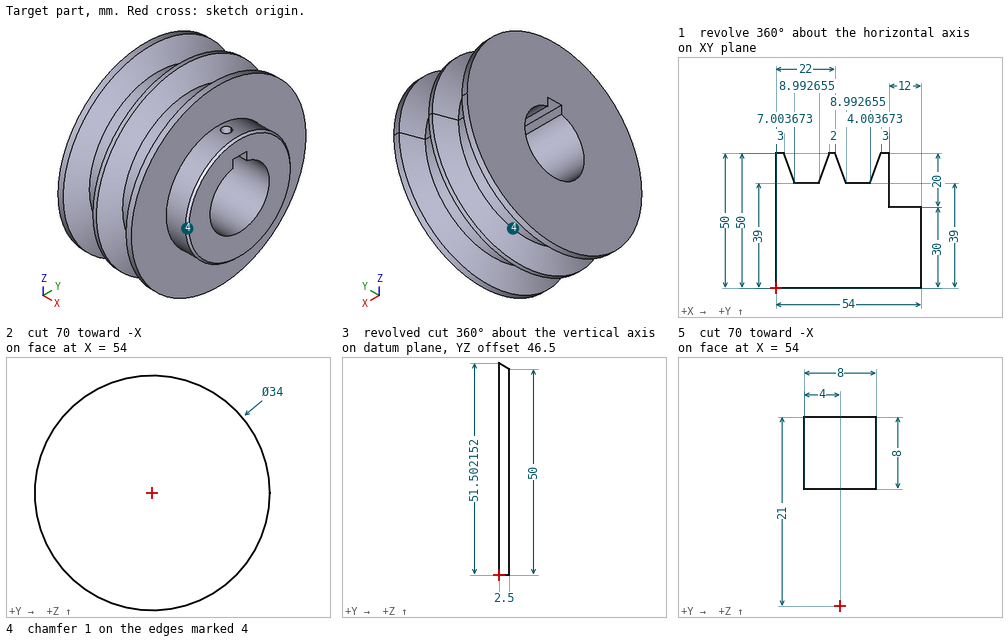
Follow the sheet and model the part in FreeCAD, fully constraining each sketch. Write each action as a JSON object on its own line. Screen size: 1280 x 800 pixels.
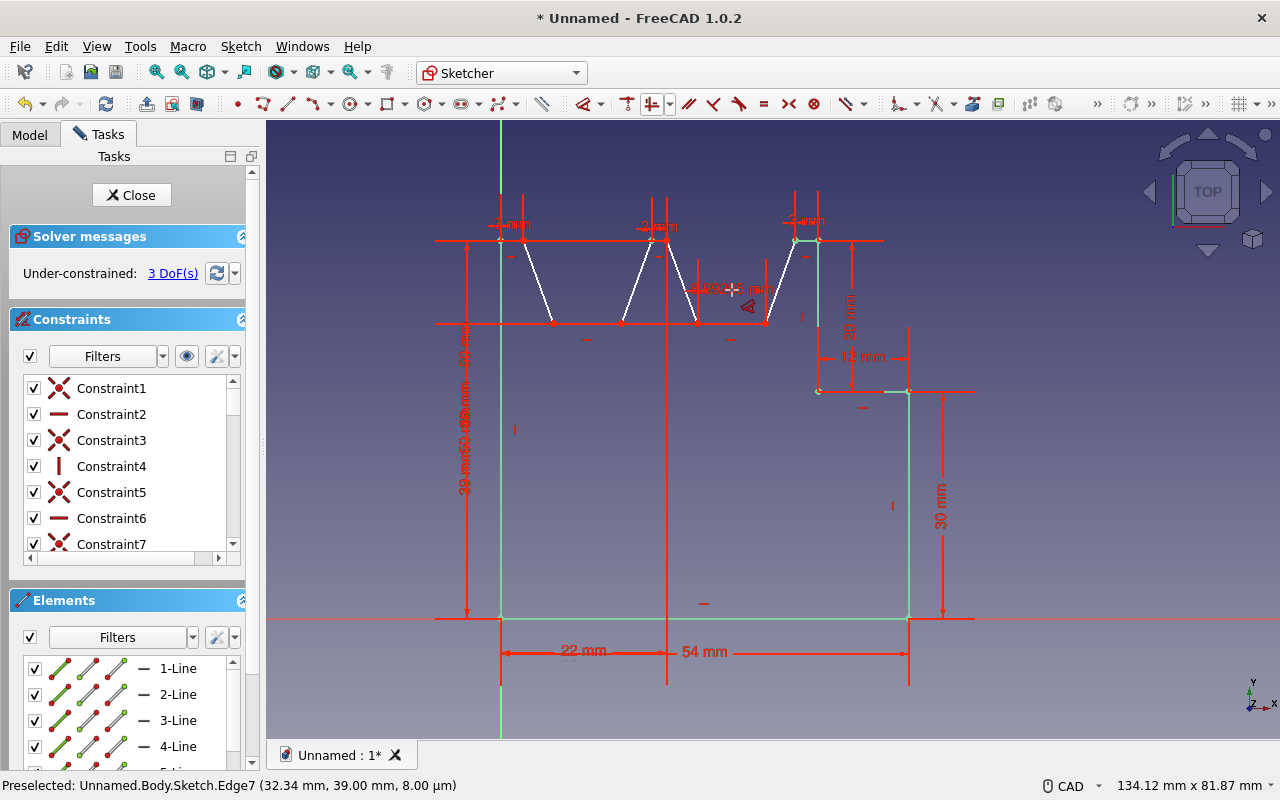
{"action": "left_click", "coordinate": [601, 324]}
{"action": "left_click", "coordinate": [588, 290]}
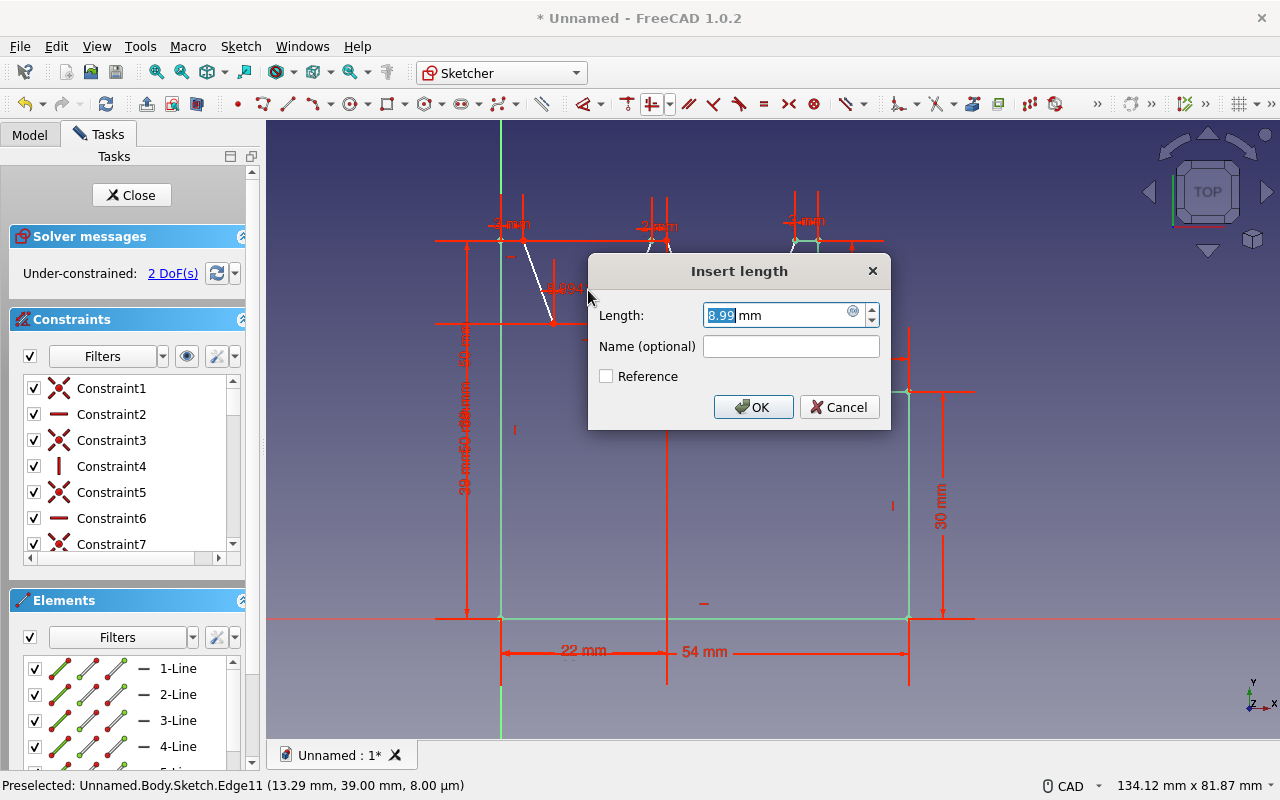
{"action": "type", "text": "8.992655"}
{"action": "key", "text": "Return"}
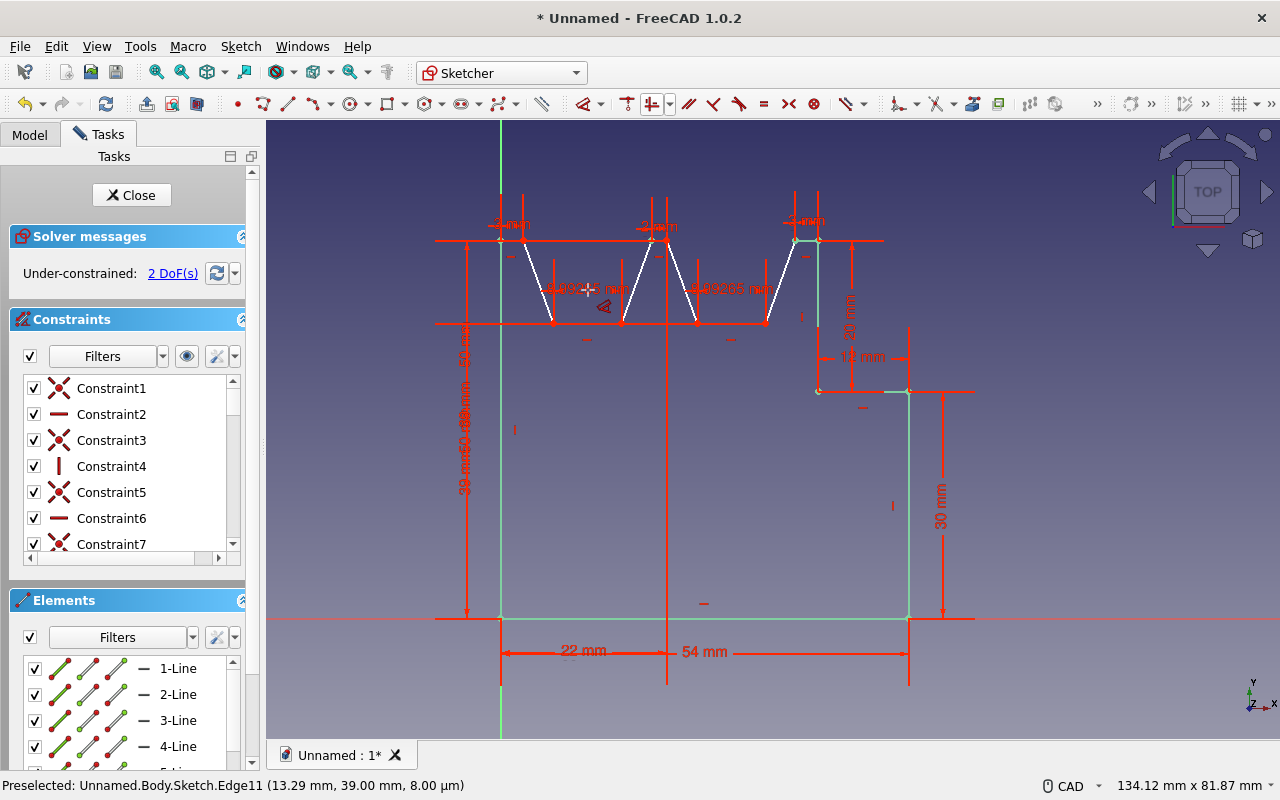
{"action": "left_click", "coordinate": [554, 324]}
{"action": "left_click", "coordinate": [515, 290]}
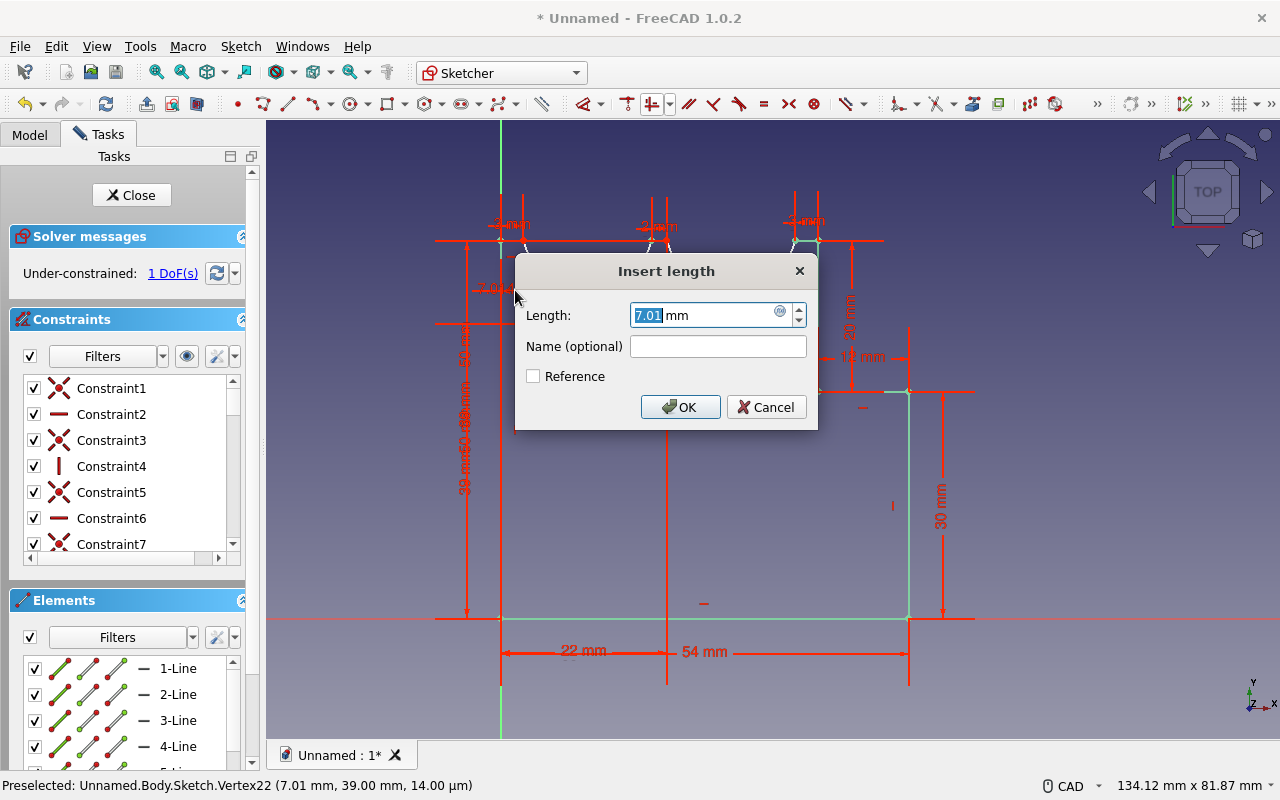
{"action": "type", "text": "7.003673"}
{"action": "key", "text": "Return"}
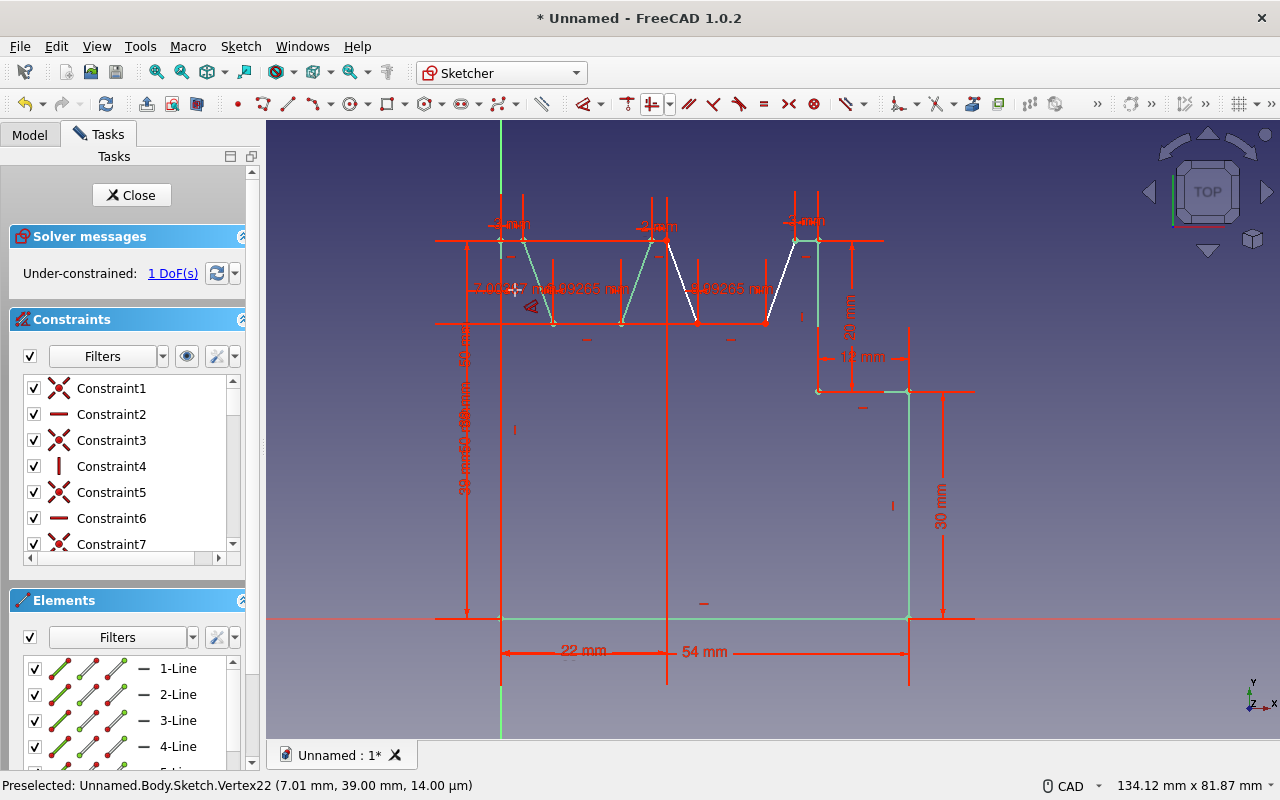
{"action": "scroll", "coordinate": [786, 266], "scroll_direction": "up", "scroll_amount": 2}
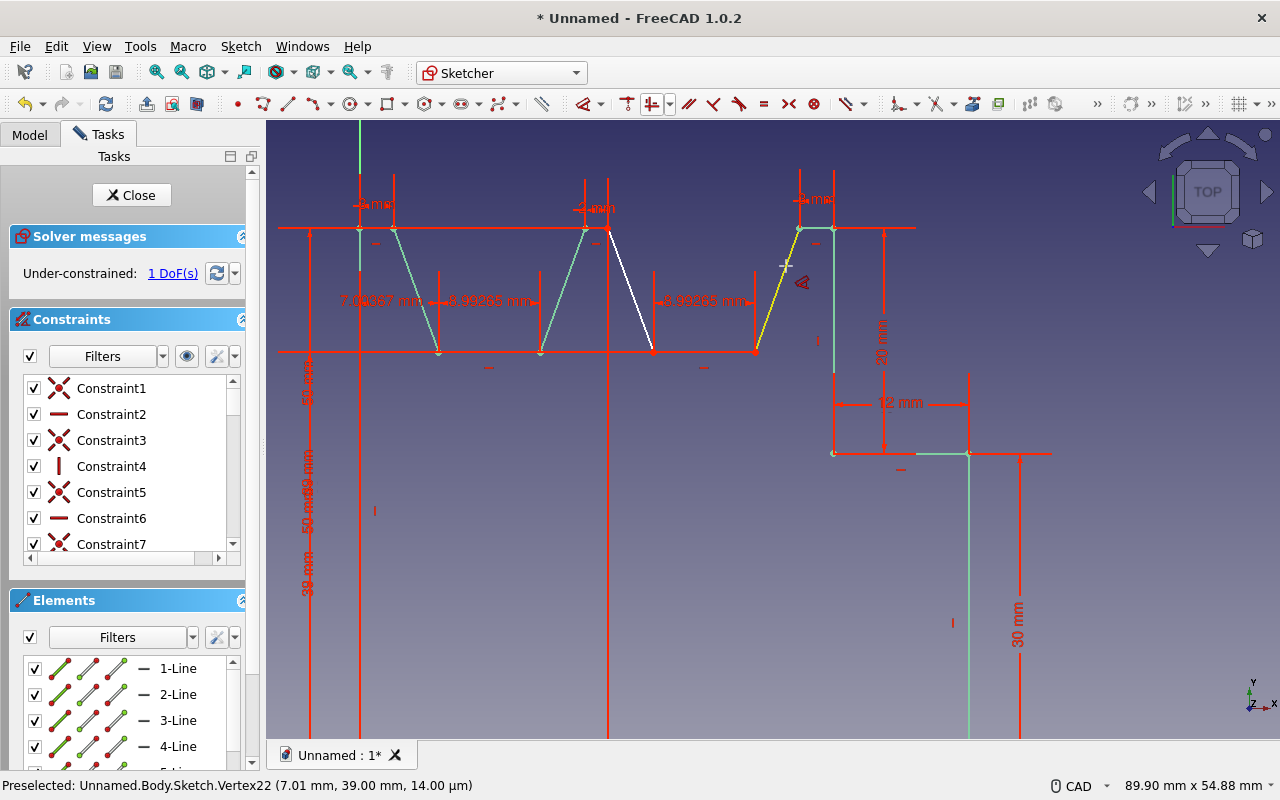
{"action": "left_click", "coordinate": [786, 265]}
{"action": "left_click", "coordinate": [777, 386]}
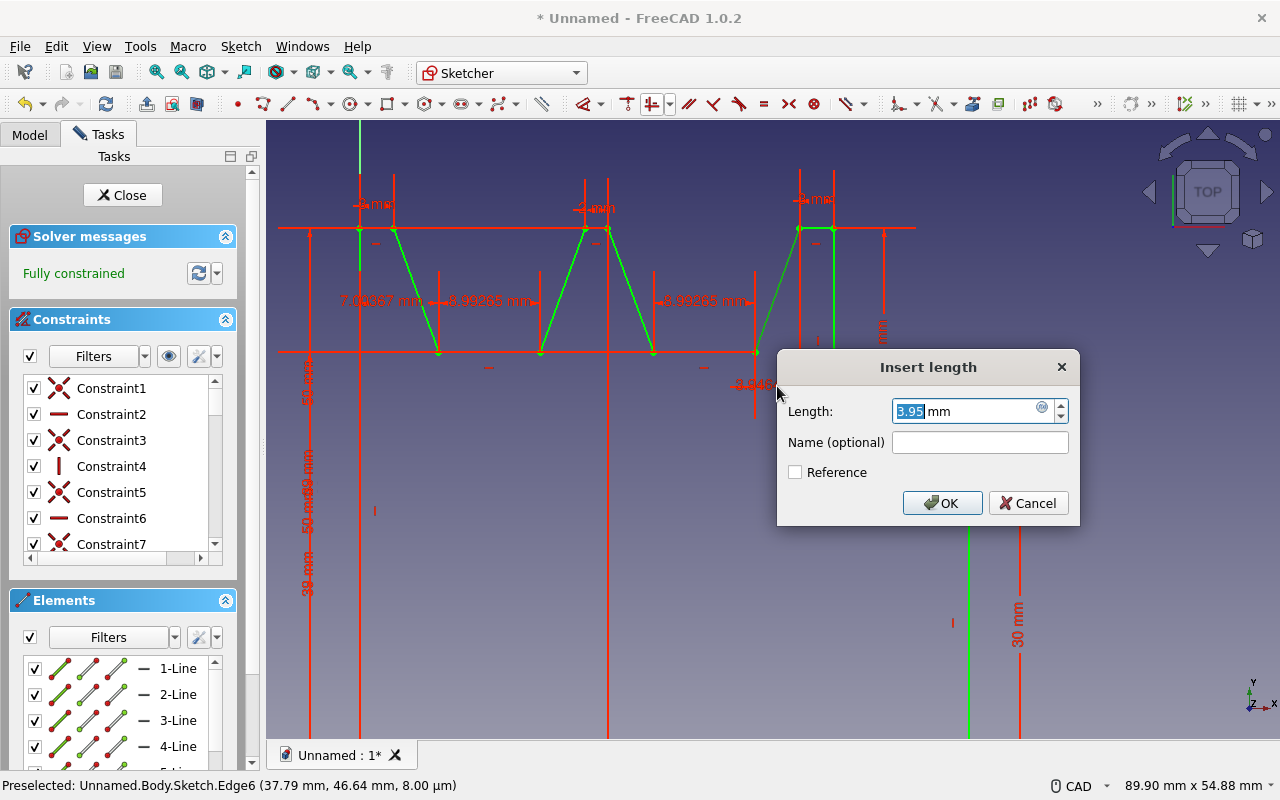
{"action": "type", "text": "4.003673"}
{"action": "key", "text": "Return"}
{"action": "key", "text": "Escape"}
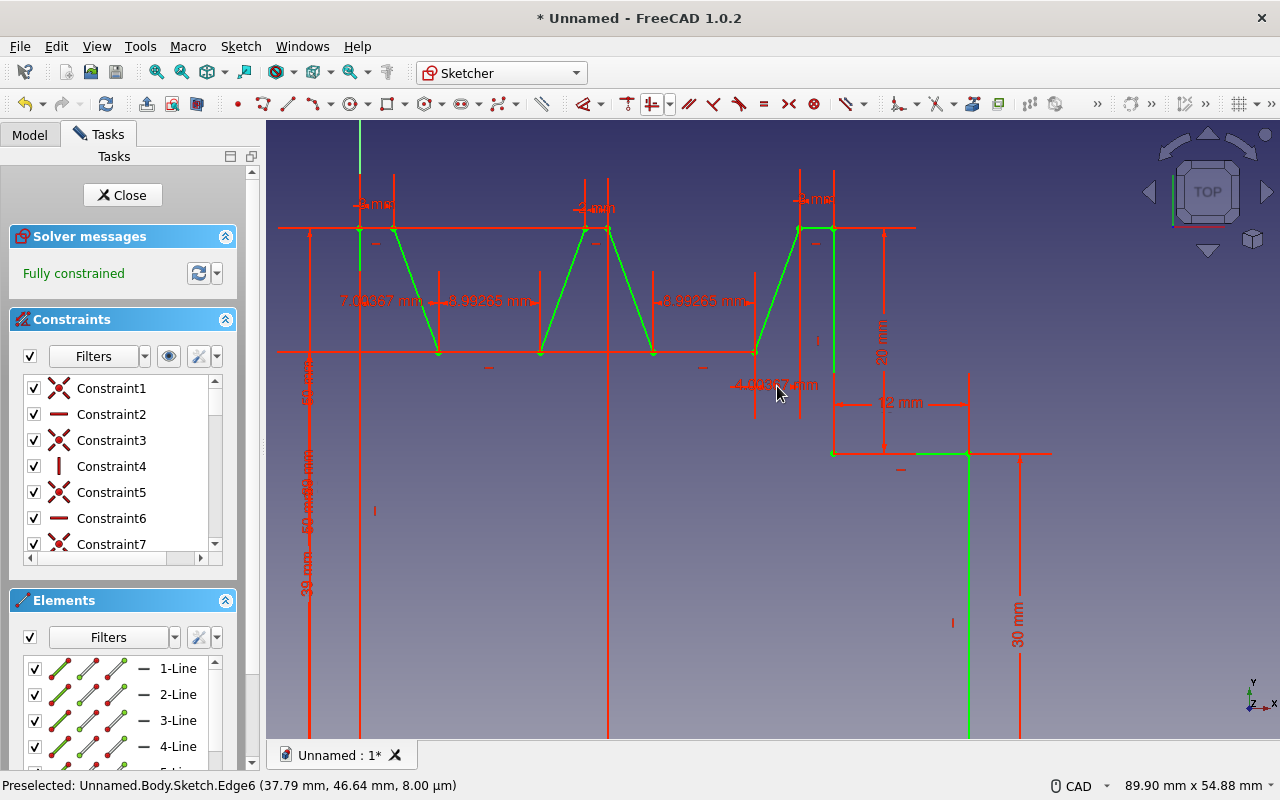
{"action": "left_click", "coordinate": [123, 195]}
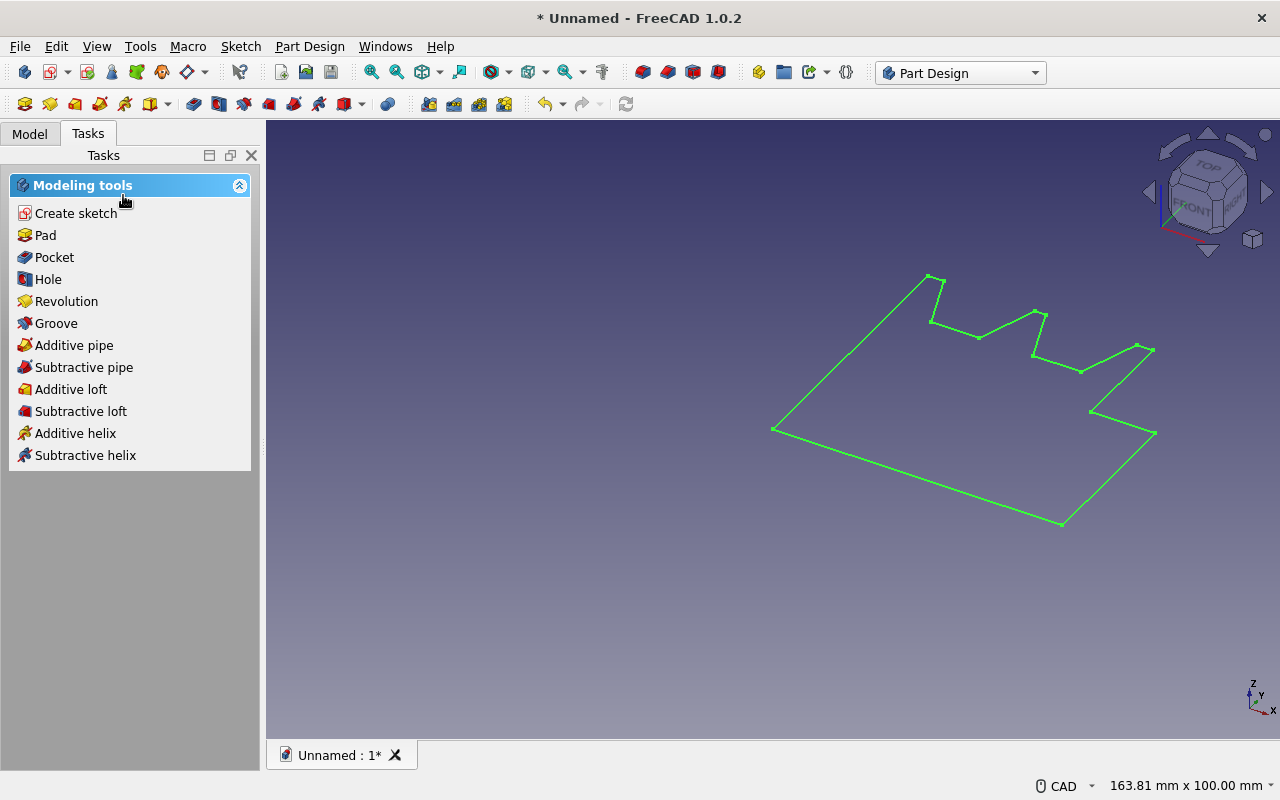
{"action": "left_click", "coordinate": [50, 104]}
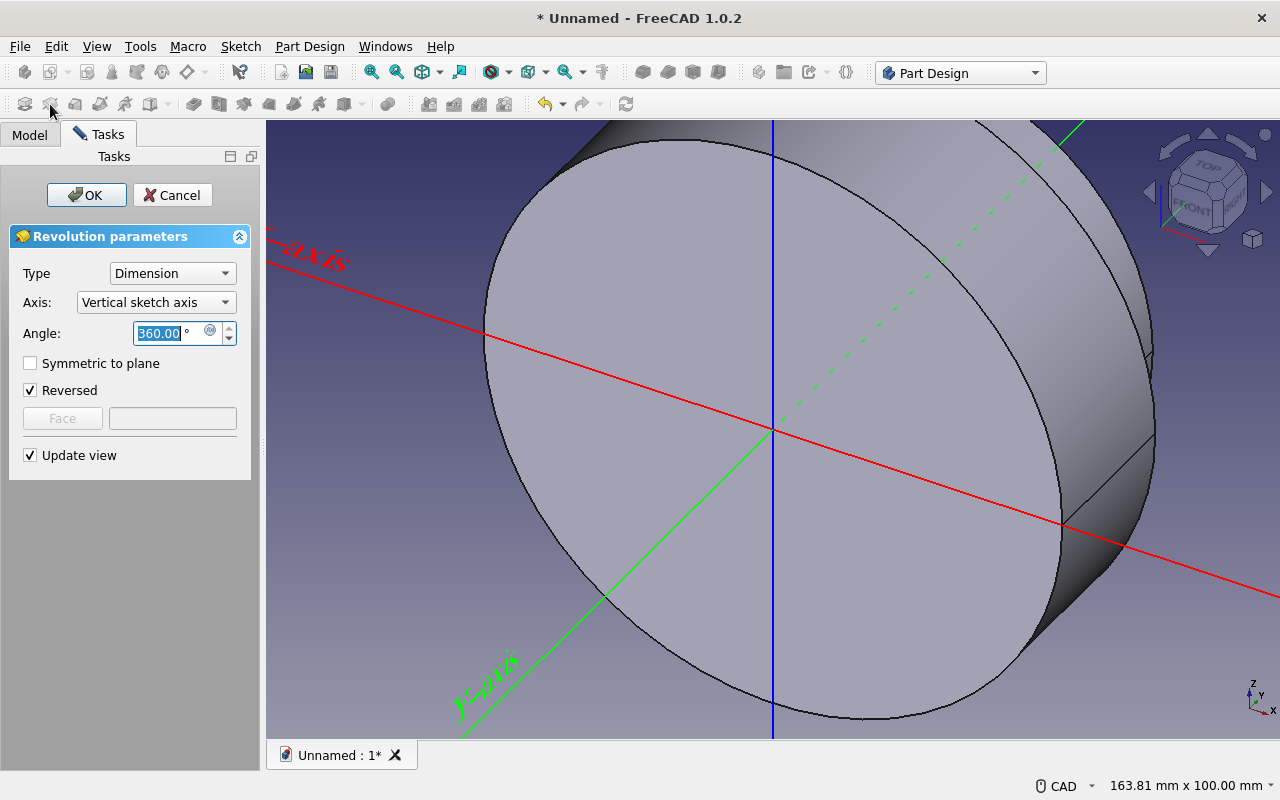
{"action": "left_click", "coordinate": [157, 302]}